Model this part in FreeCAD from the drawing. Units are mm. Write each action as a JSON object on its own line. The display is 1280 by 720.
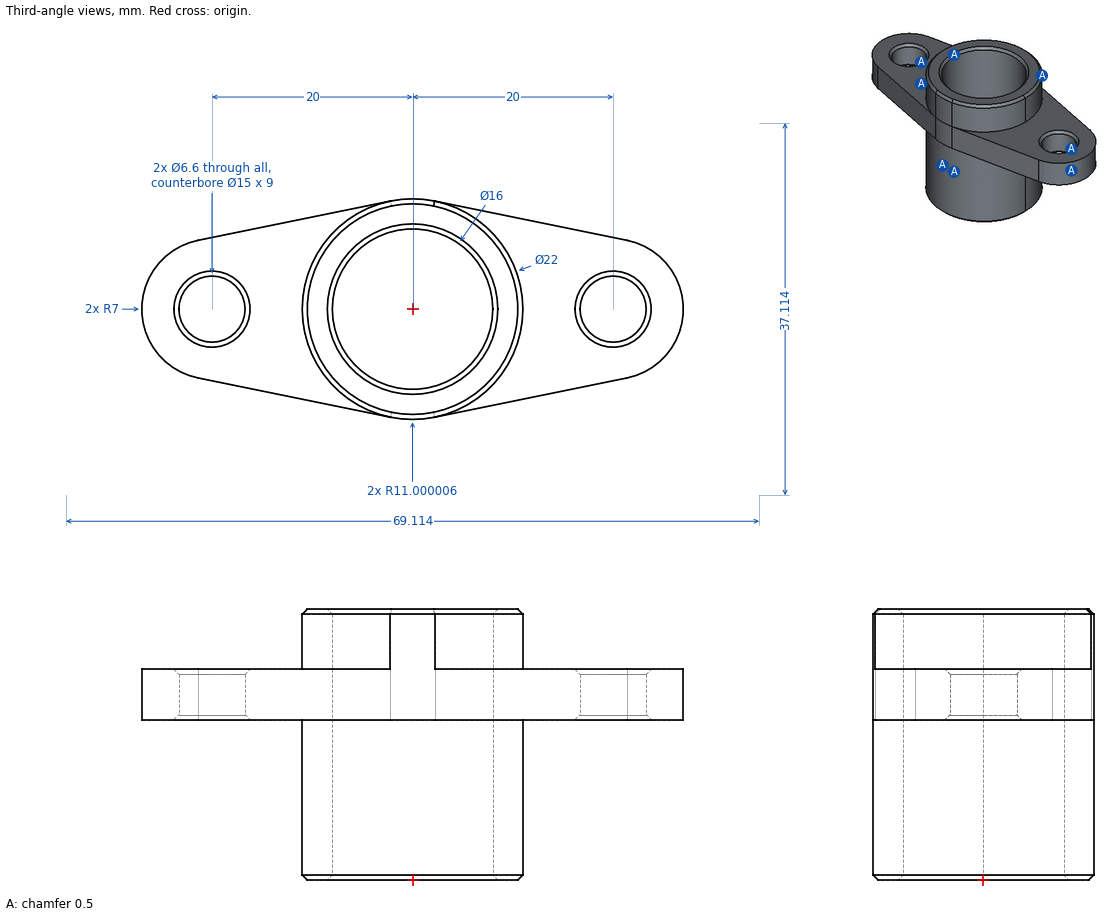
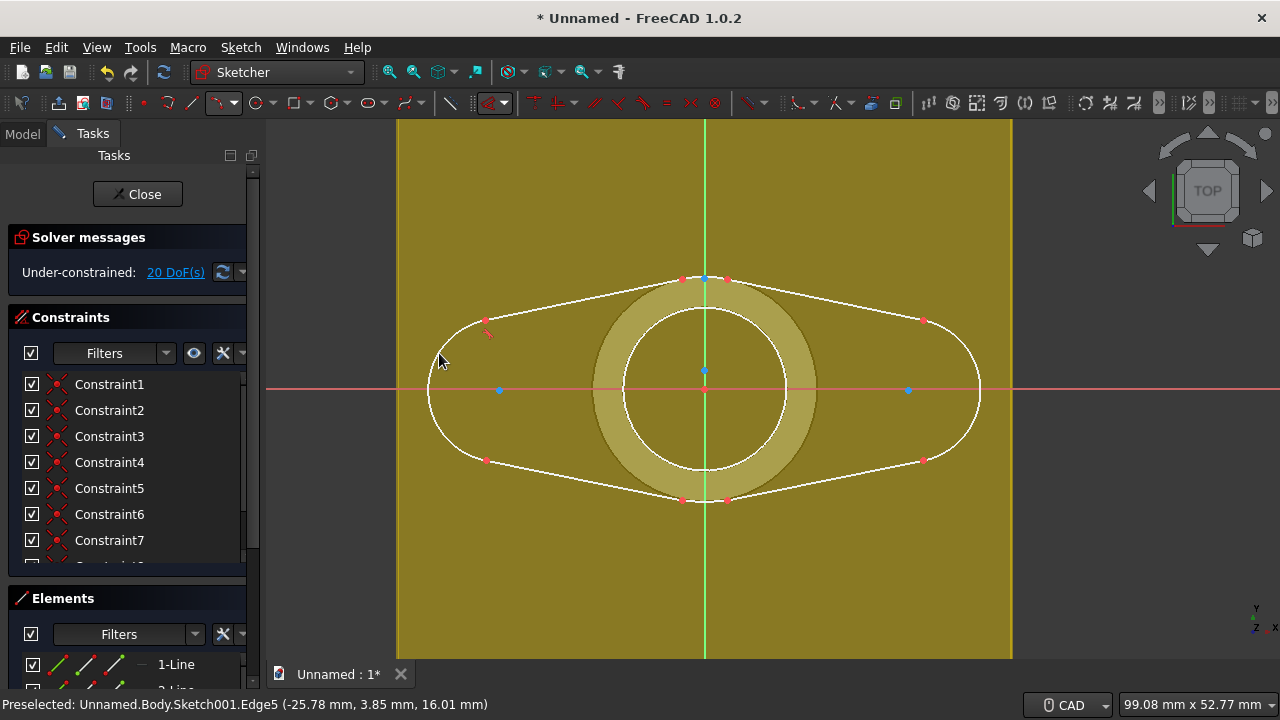
{"action": "left_click", "coordinate": [623, 292]}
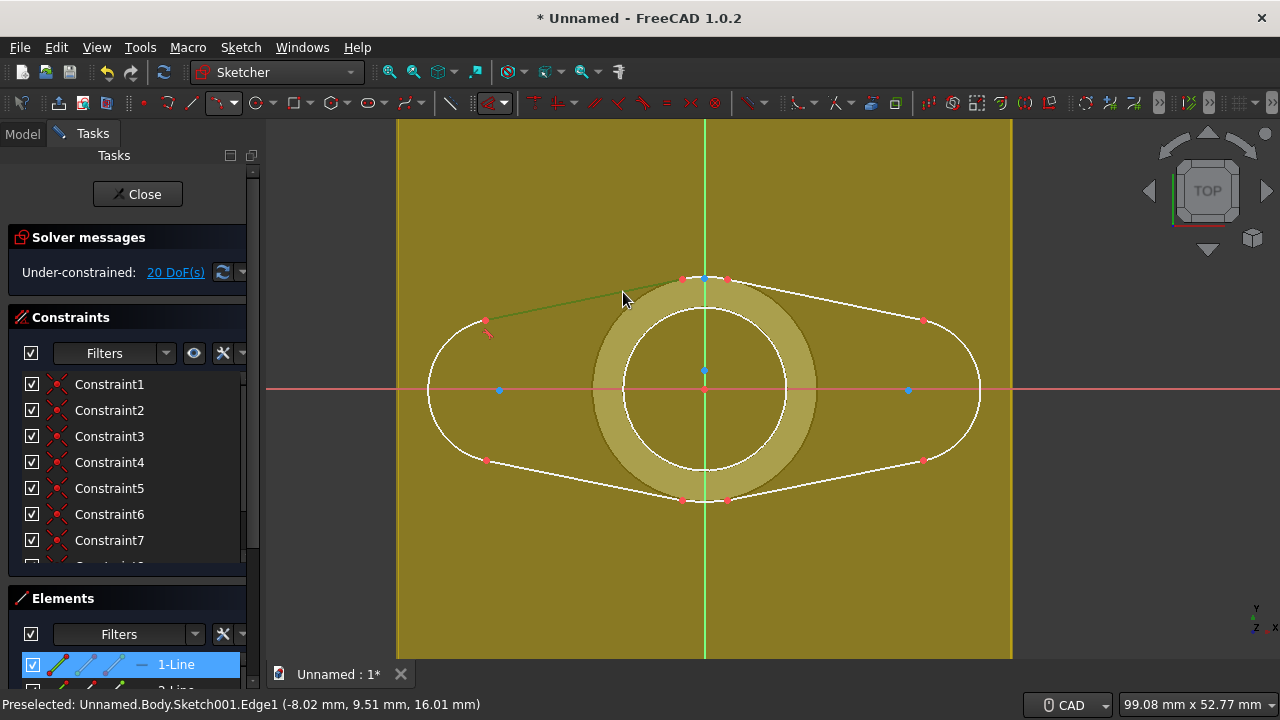
{"action": "scroll", "coordinate": [696, 277], "scroll_direction": "up", "scroll_amount": 3}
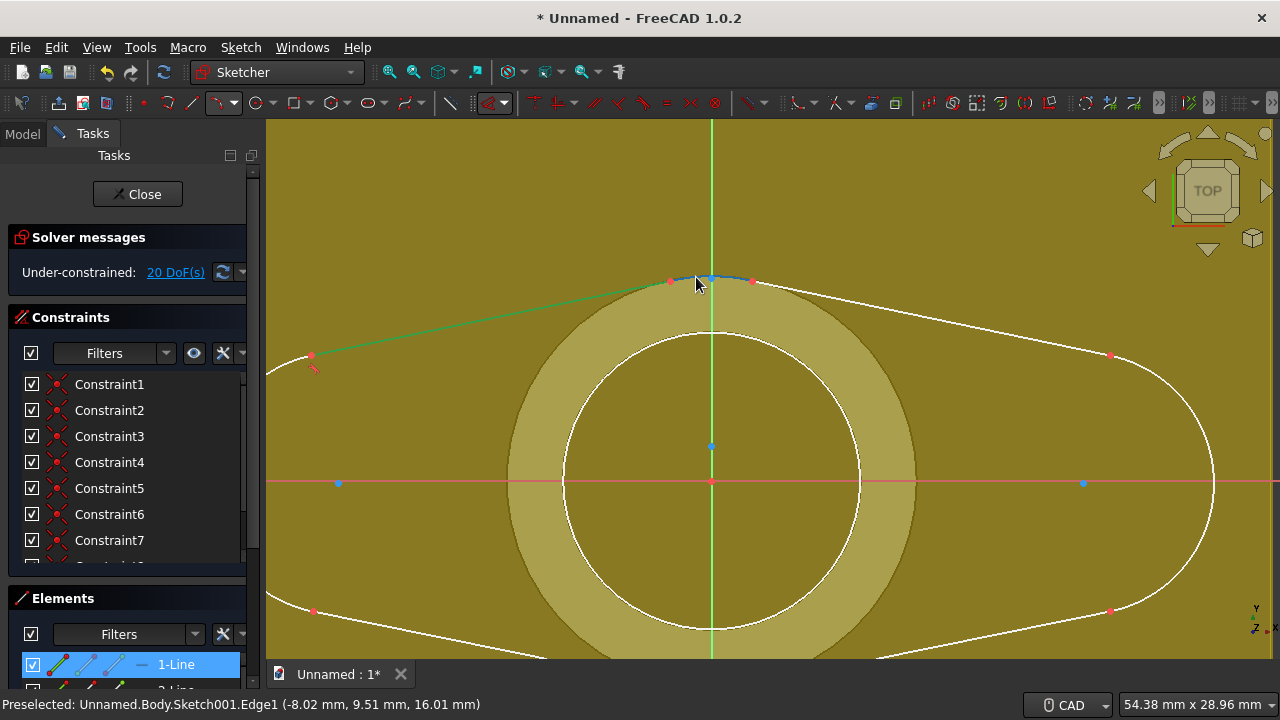
{"action": "left_click", "coordinate": [695, 277]}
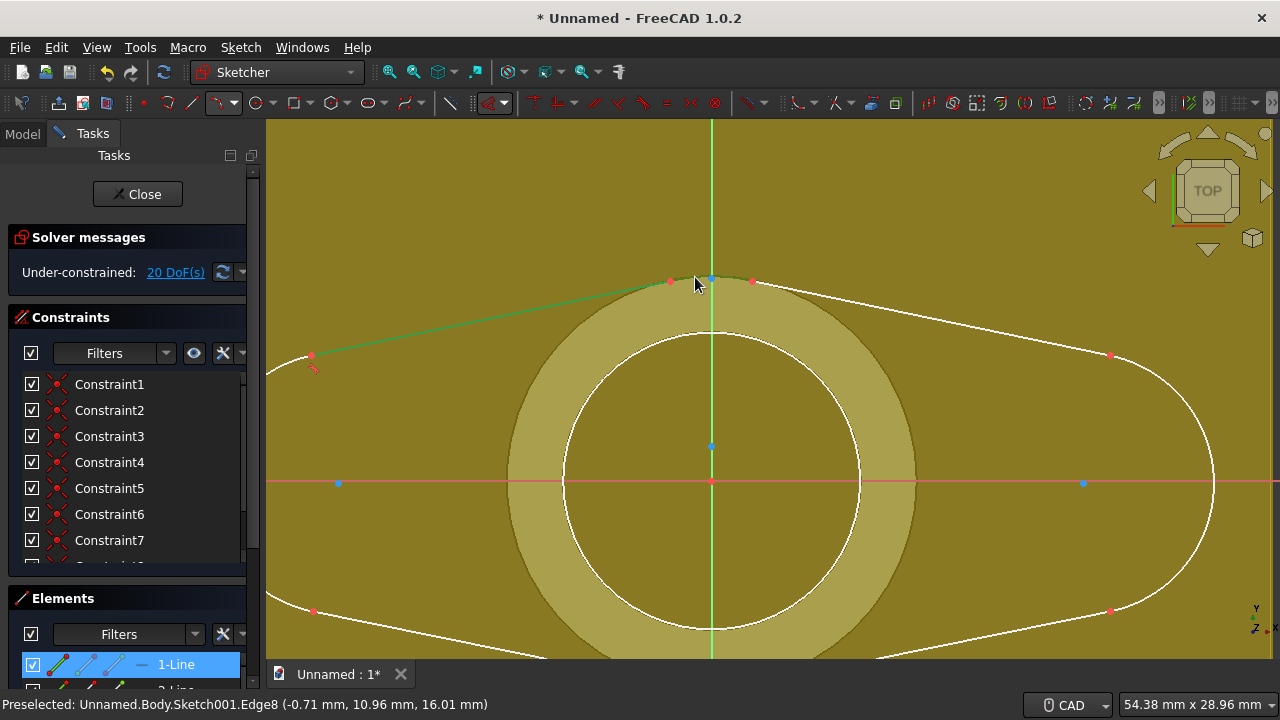
{"action": "left_click", "coordinate": [644, 104]}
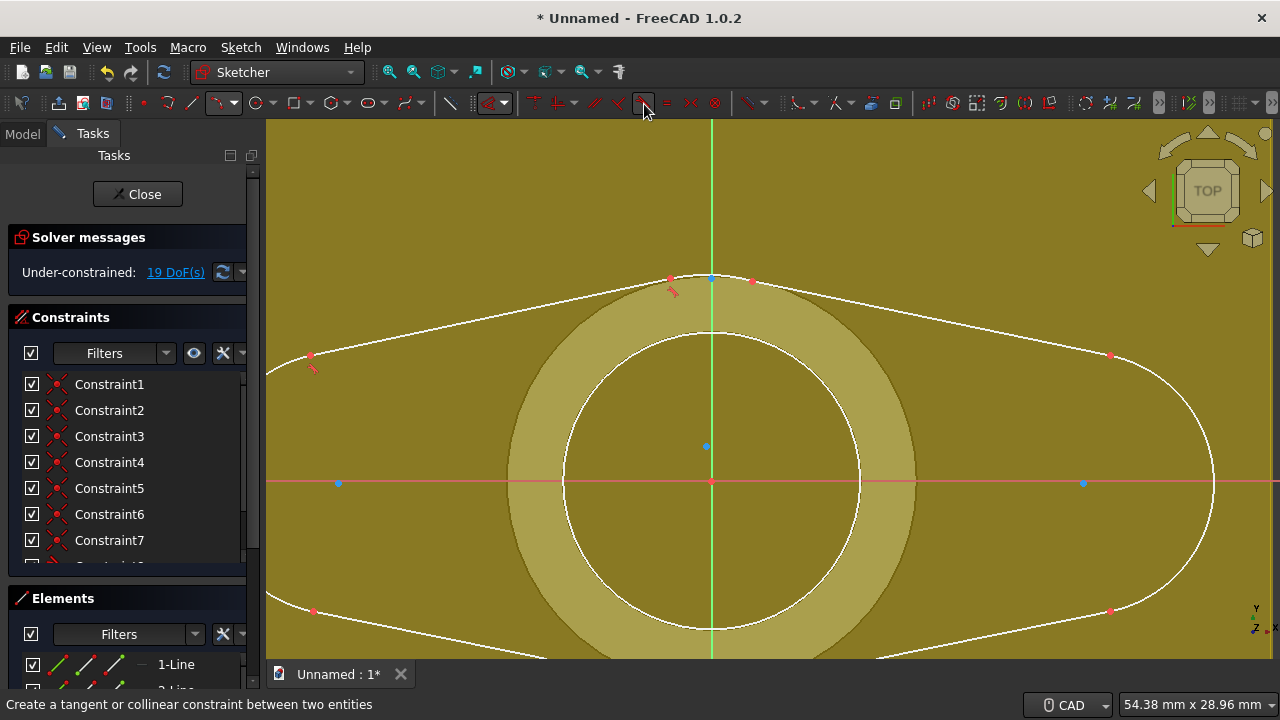
{"action": "left_click", "coordinate": [385, 626]}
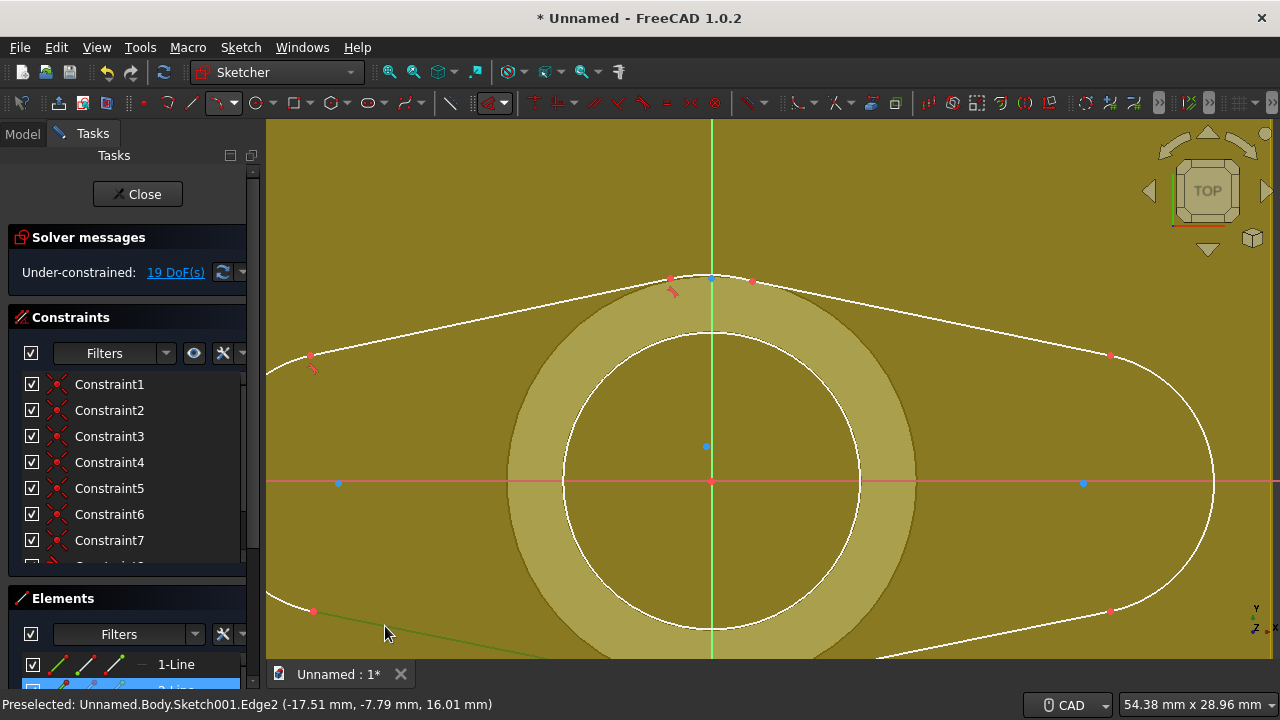
{"action": "scroll", "coordinate": [696, 277], "scroll_direction": "down", "scroll_amount": 3}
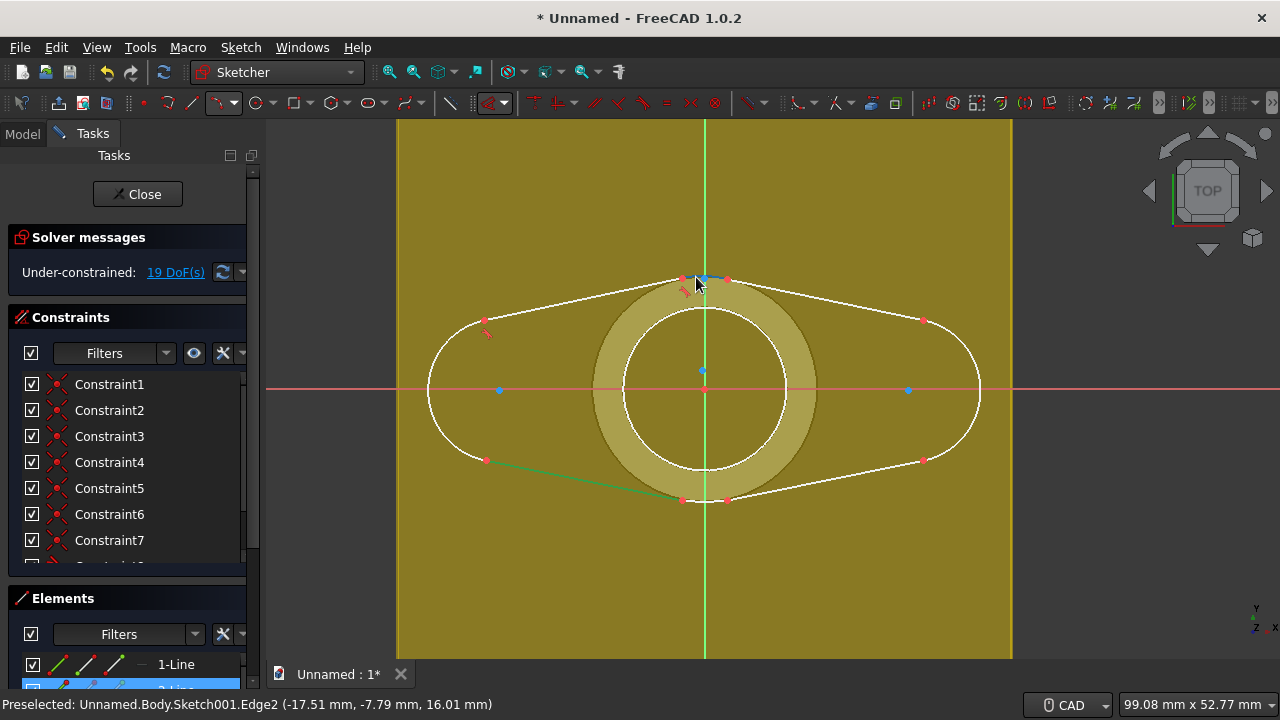
{"action": "left_click", "coordinate": [438, 354]}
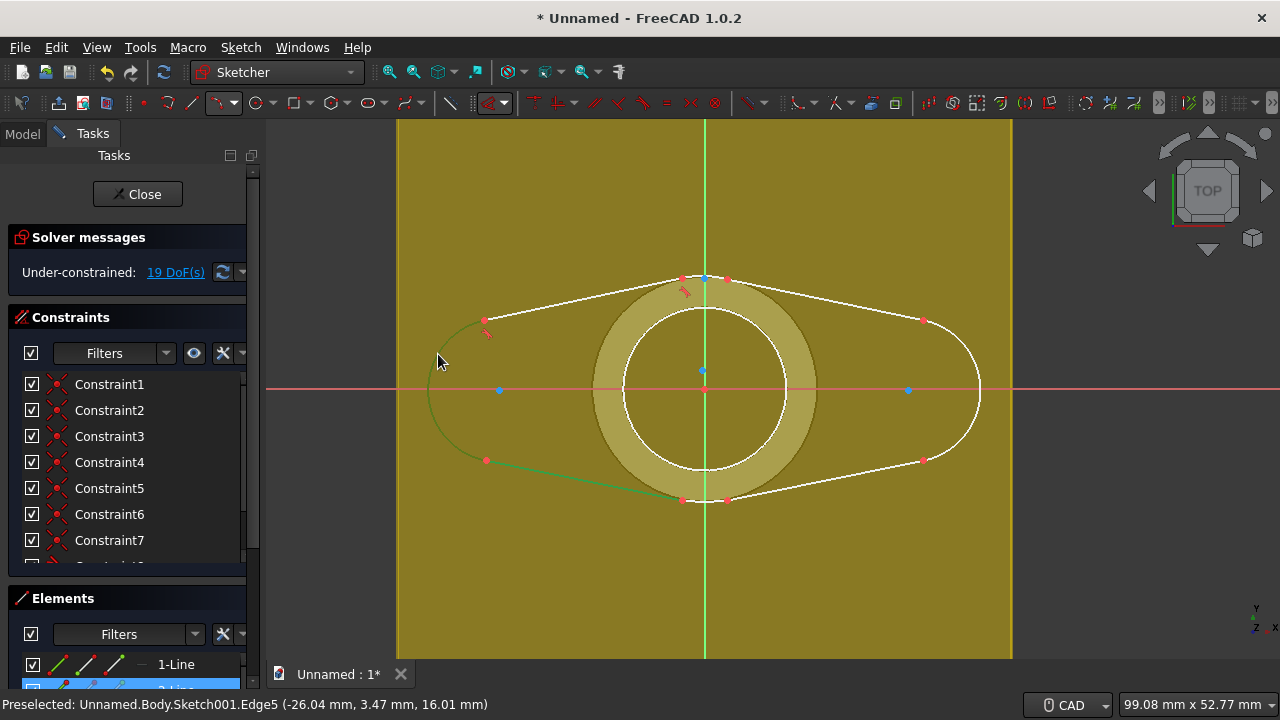
{"action": "left_click", "coordinate": [644, 104]}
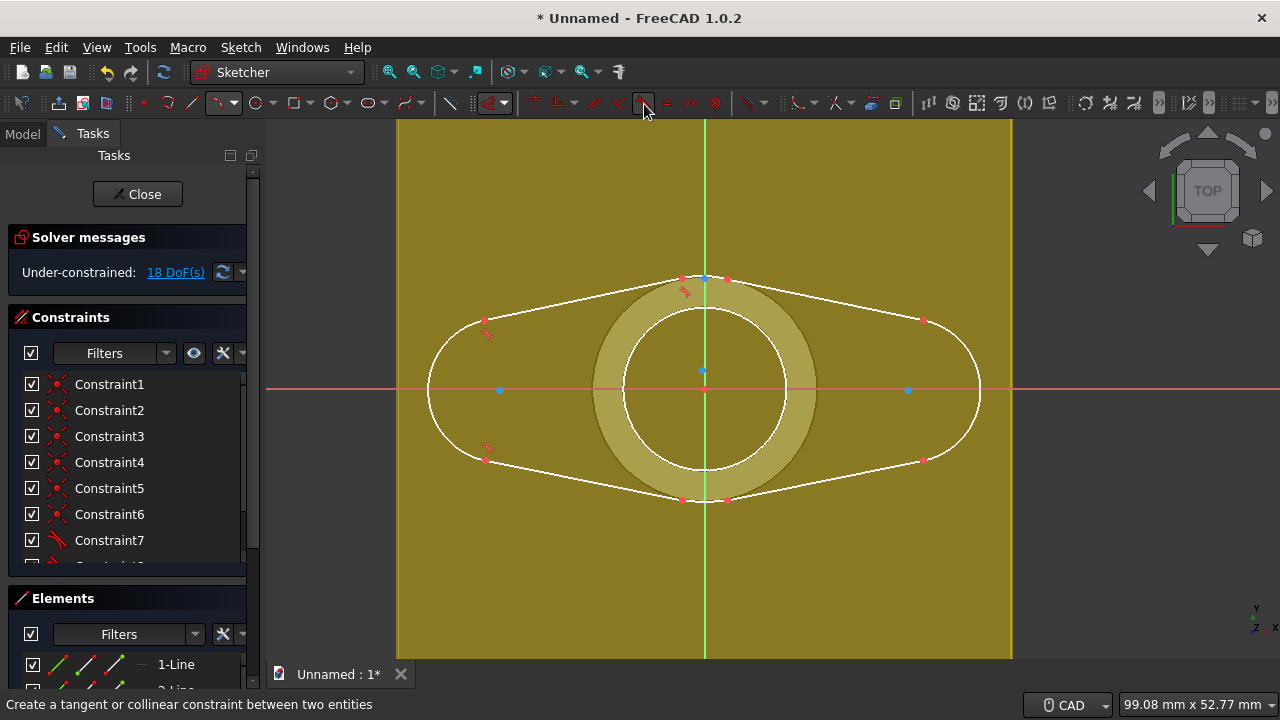
{"action": "left_click", "coordinate": [545, 473]}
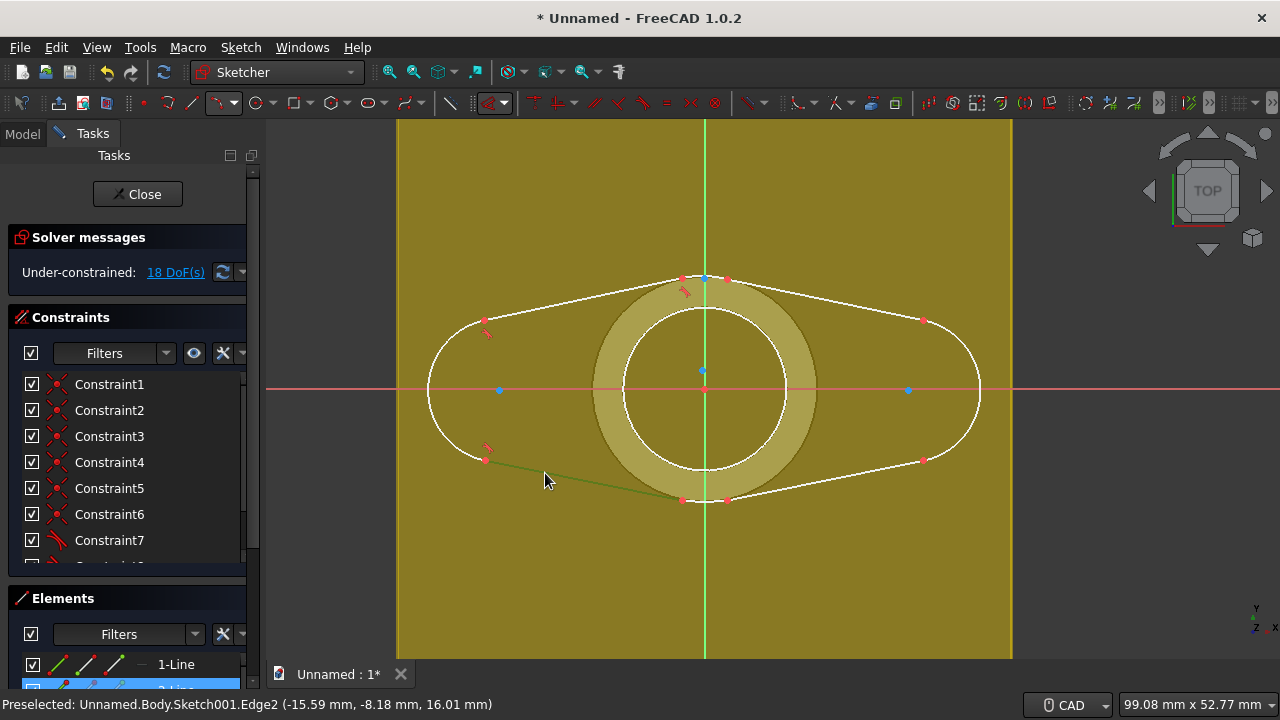
{"action": "scroll", "coordinate": [696, 502], "scroll_direction": "up", "scroll_amount": 3}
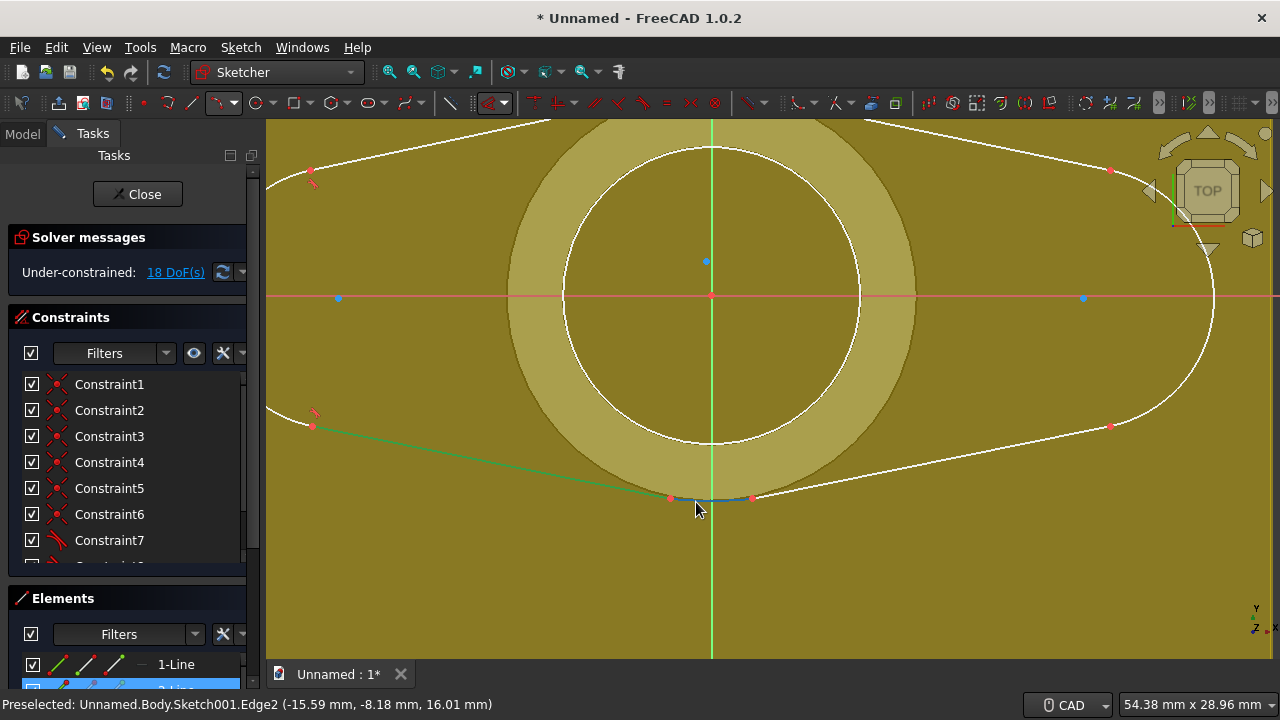
{"action": "left_click", "coordinate": [695, 501]}